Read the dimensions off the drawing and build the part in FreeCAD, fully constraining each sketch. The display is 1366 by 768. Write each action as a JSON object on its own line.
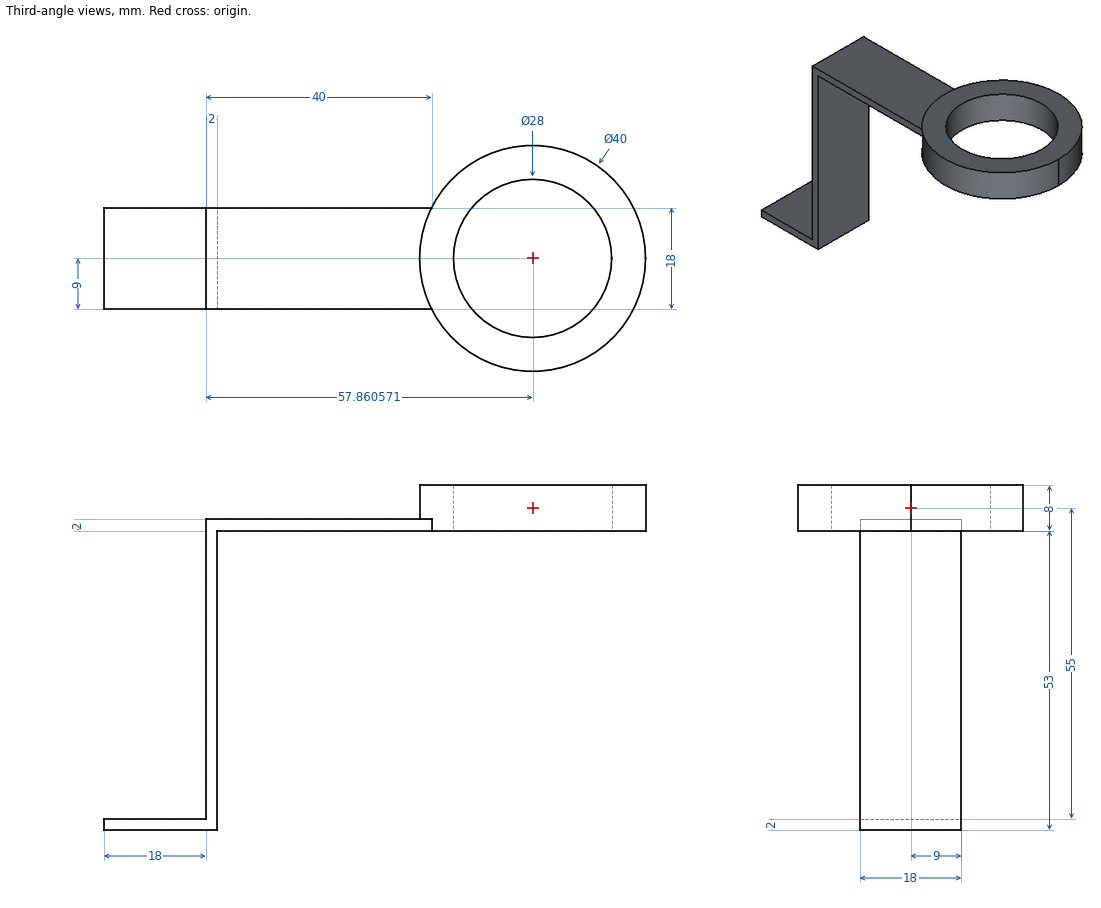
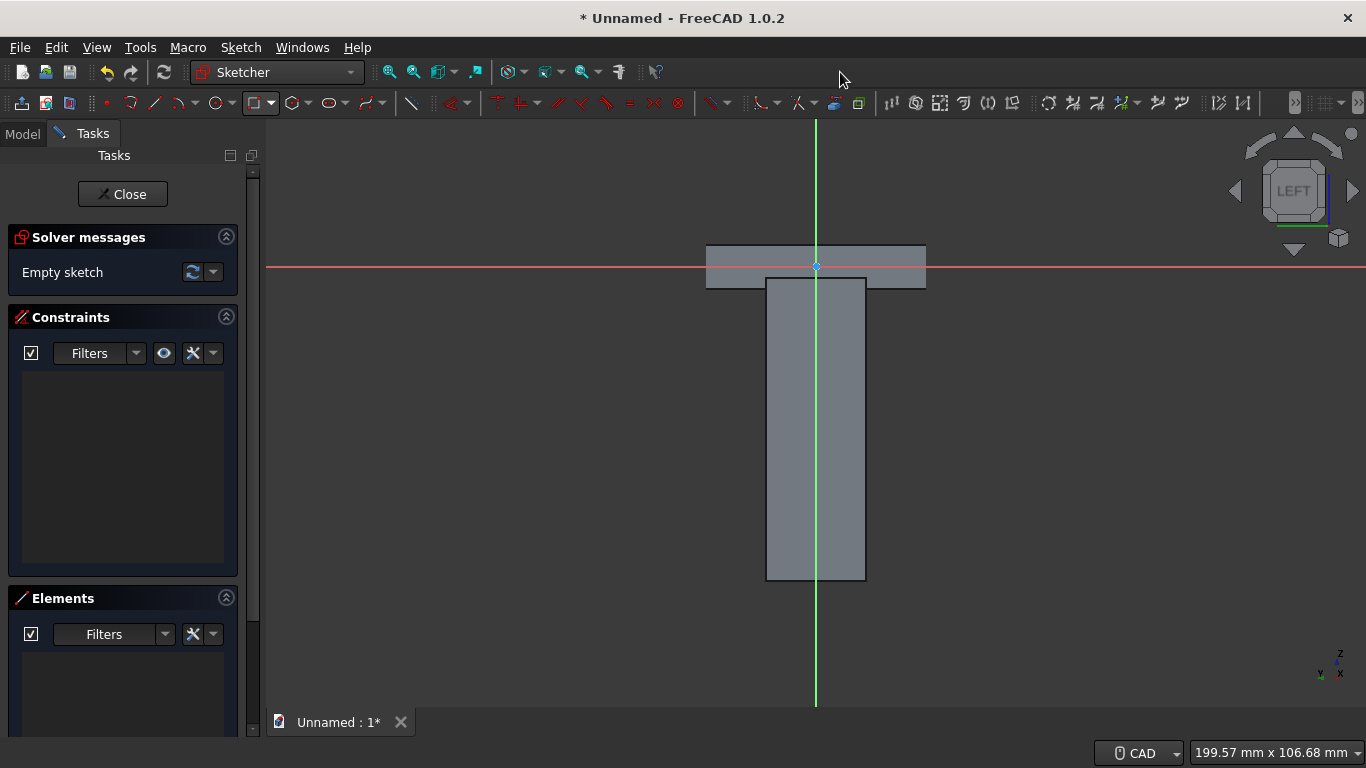
{"action": "scroll", "coordinate": [830, 608], "scroll_direction": "up", "scroll_amount": 9}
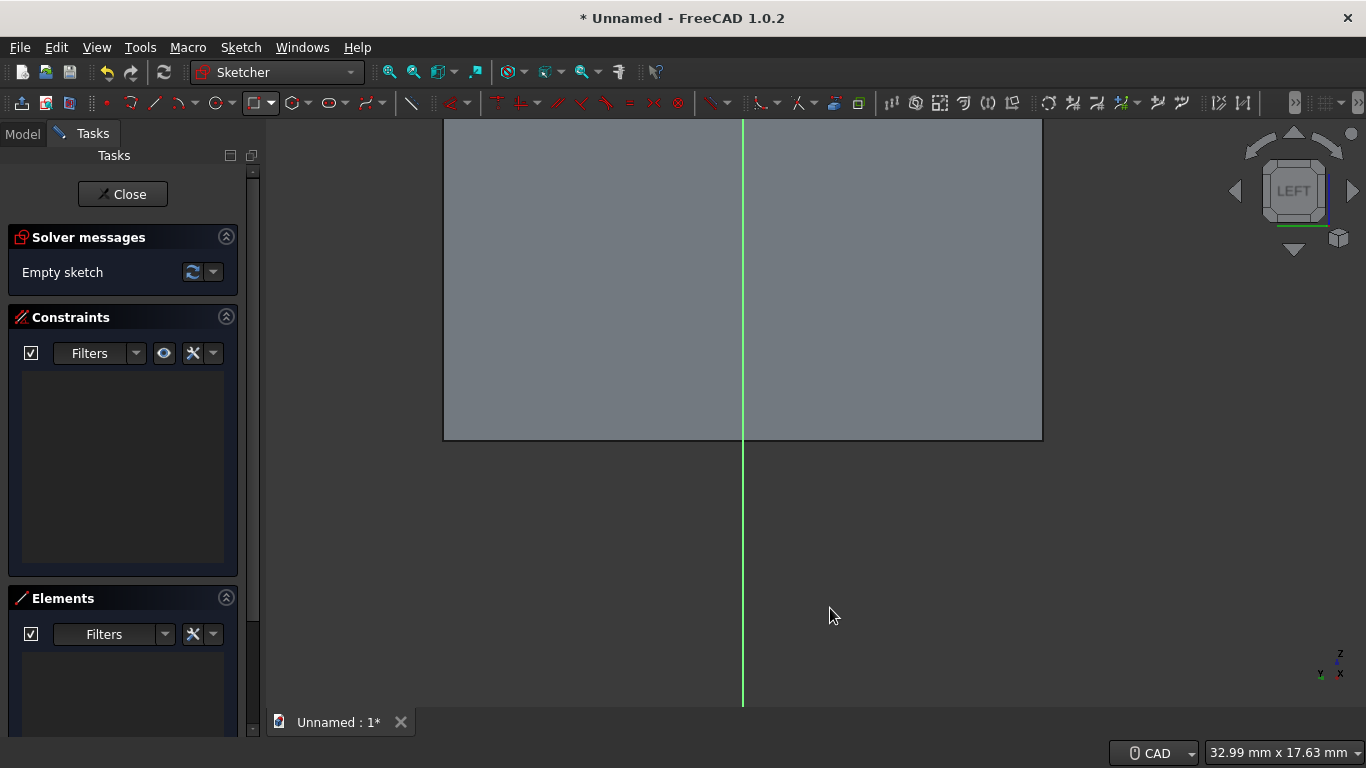
{"action": "left_click", "coordinate": [254, 104]}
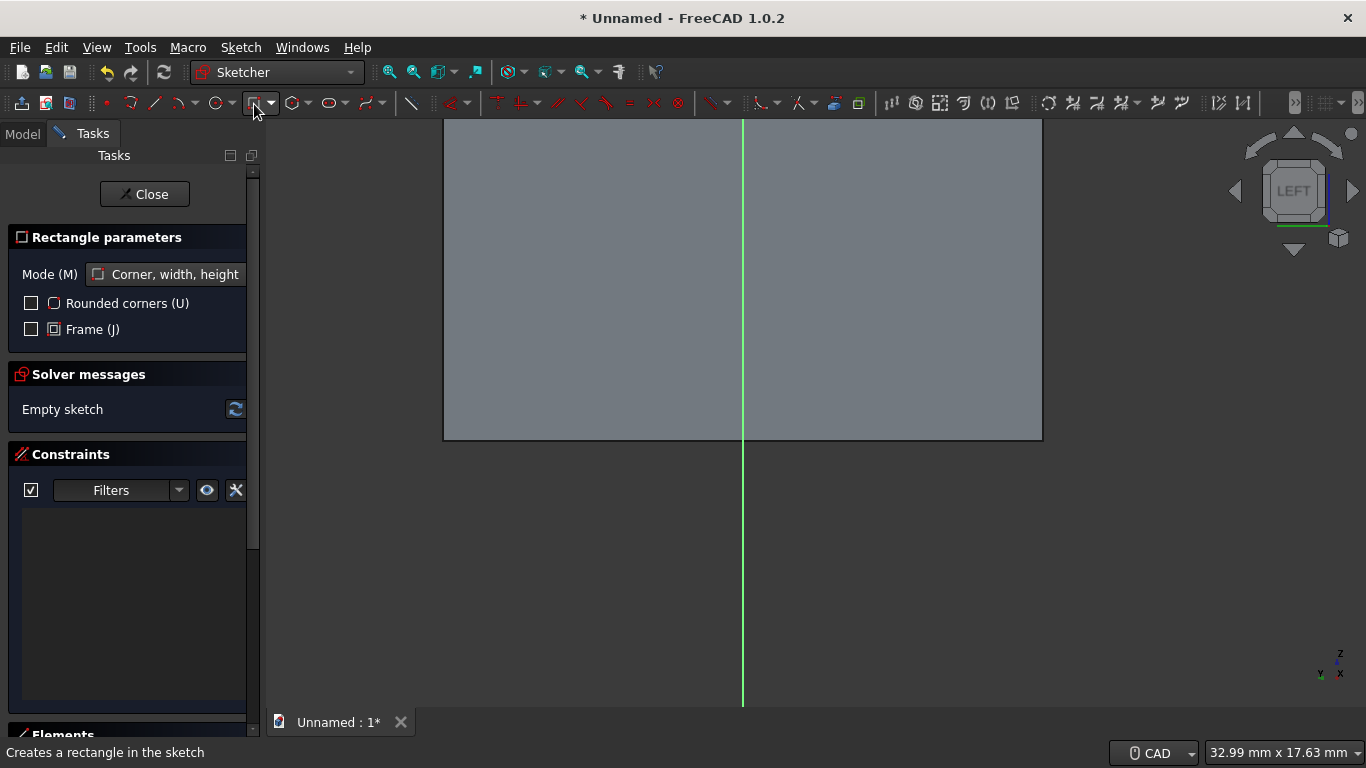
{"action": "left_click", "coordinate": [443, 374]}
{"action": "mouse_move", "coordinate": [1043, 441]}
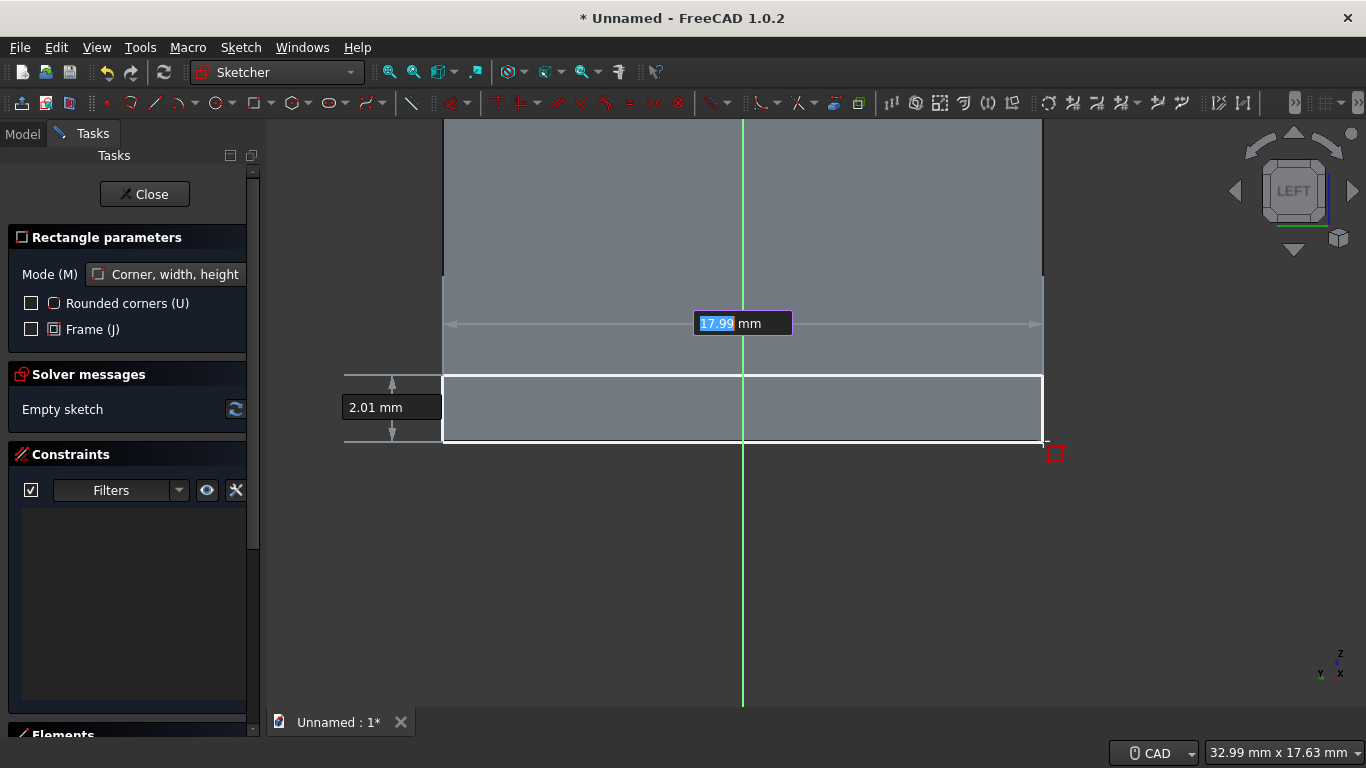
{"action": "type", "text": "18"}
{"action": "key", "text": "Tab"}
{"action": "type", "text": "2"}
{"action": "key", "text": "Return"}
{"action": "key", "text": "Escape"}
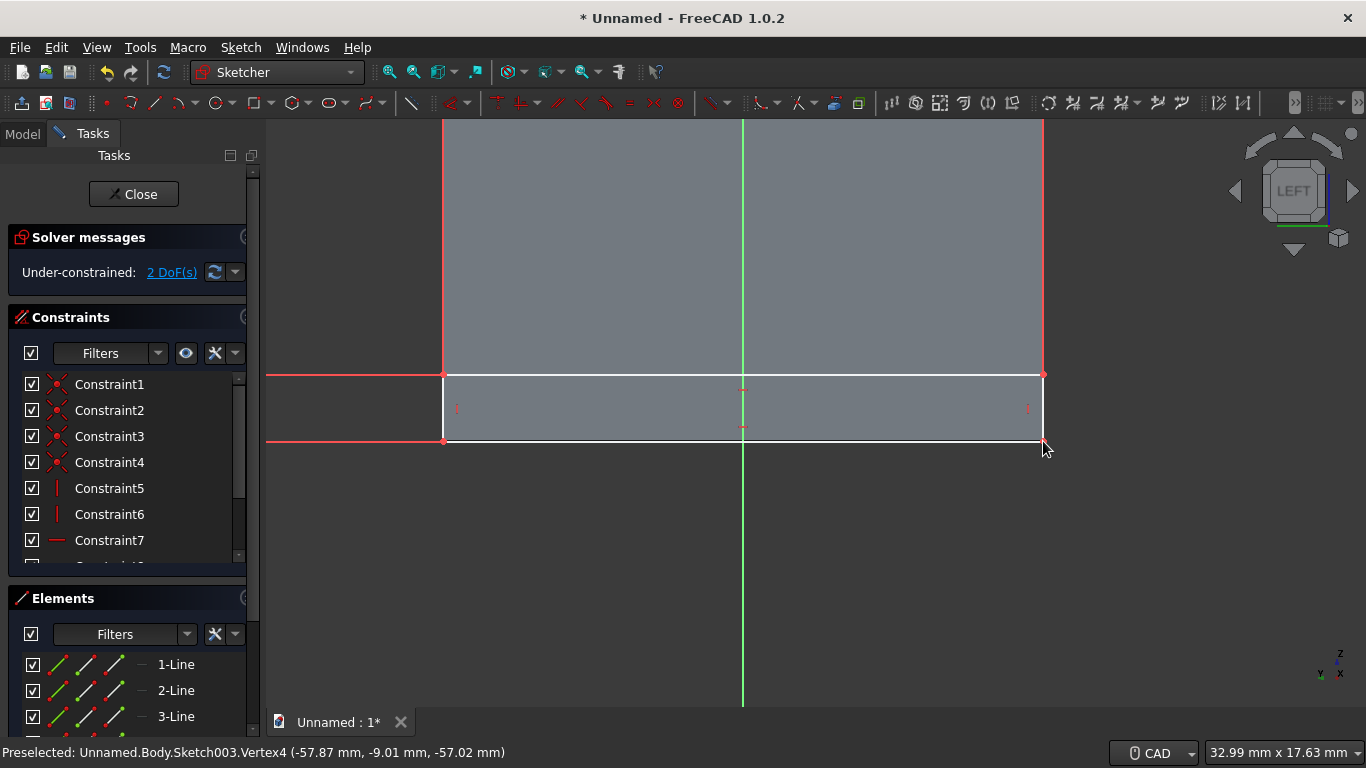
{"action": "left_click", "coordinate": [450, 104]}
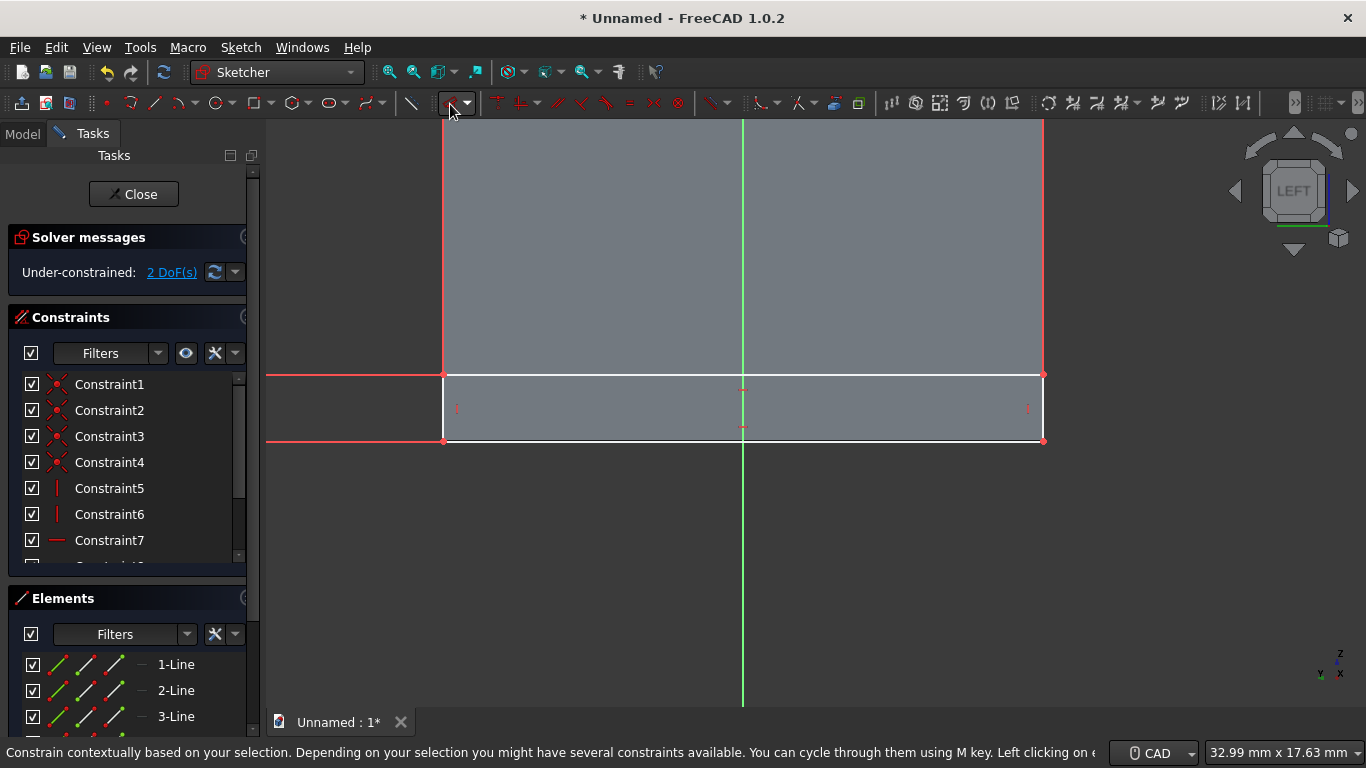
{"action": "left_click", "coordinate": [443, 375]}
{"action": "left_click", "coordinate": [593, 409]}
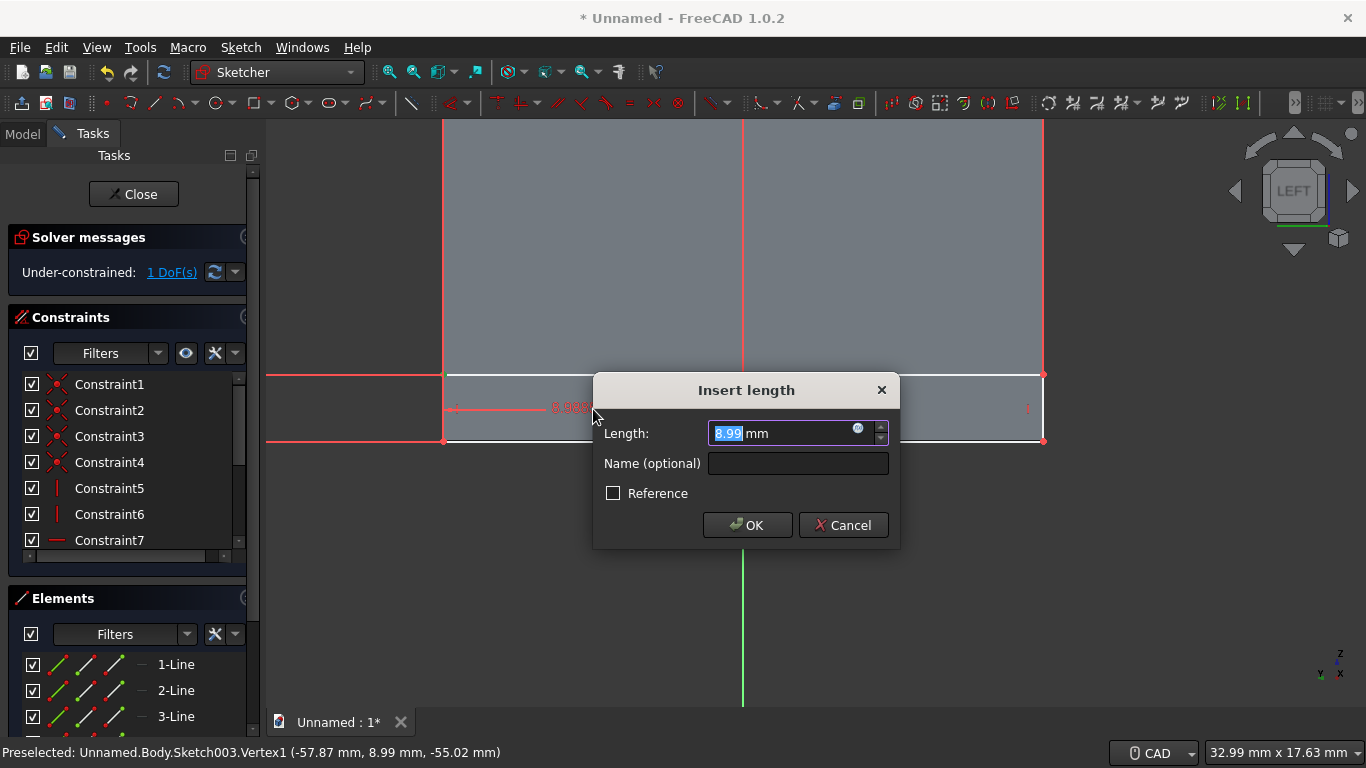
{"action": "type", "text": "9"}
{"action": "key", "text": "Return"}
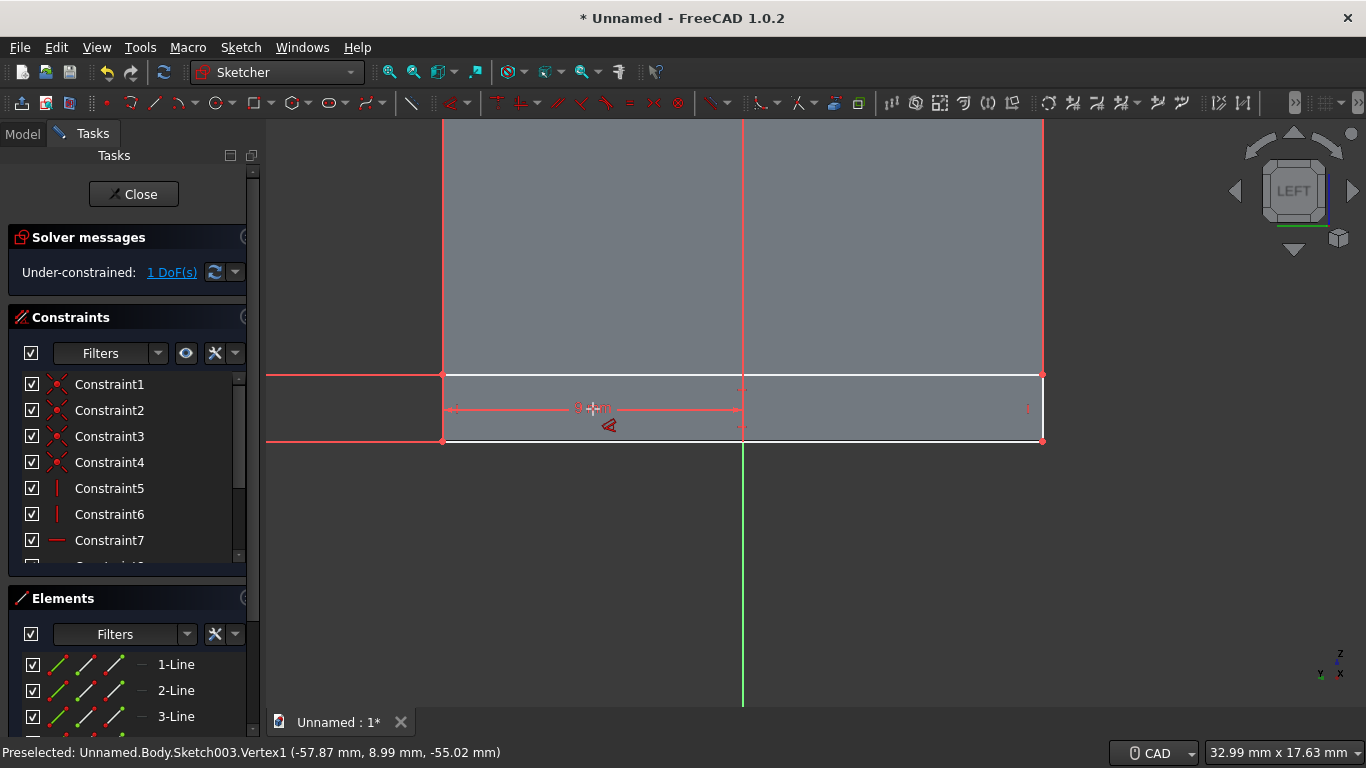
{"action": "left_click", "coordinate": [443, 375]}
{"action": "left_click", "coordinate": [409, 261]}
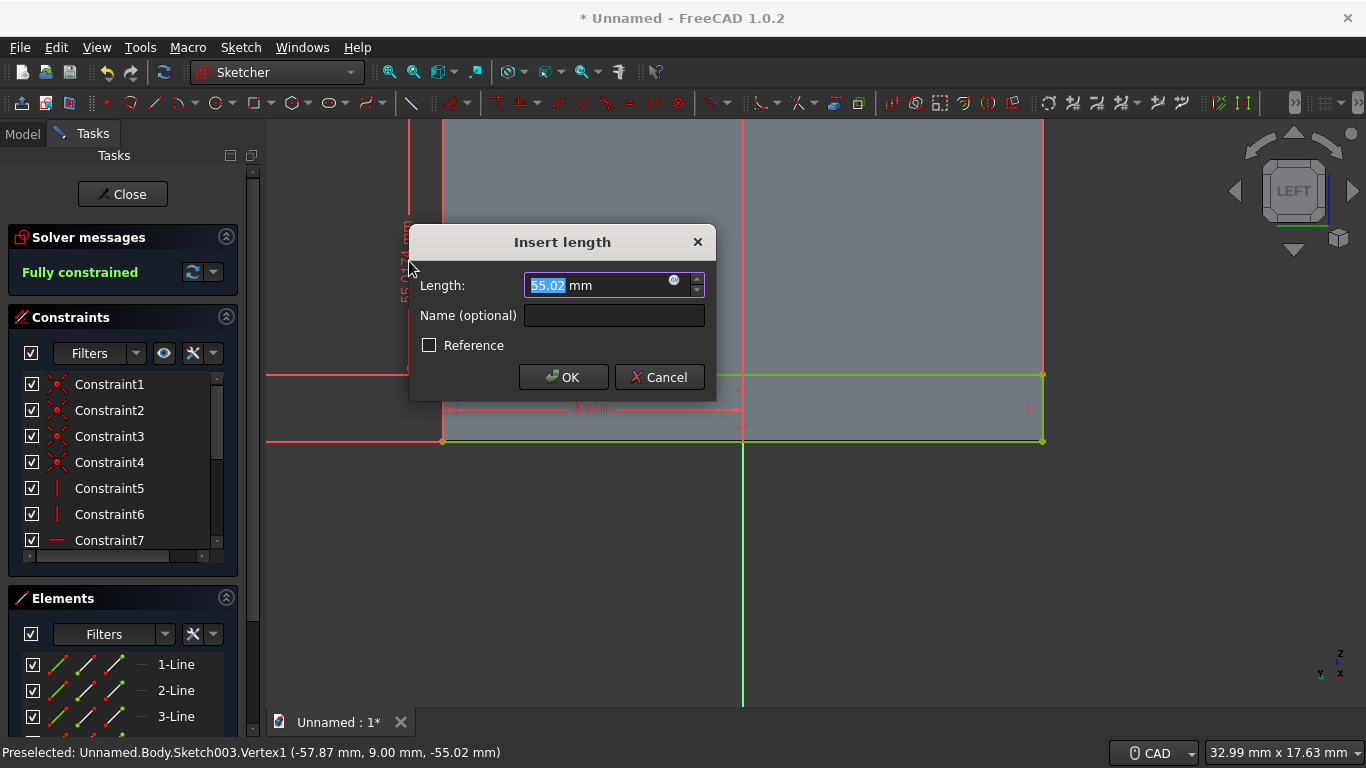
{"action": "type", "text": "55"}
{"action": "key", "text": "Return"}
{"action": "key", "text": "Escape"}